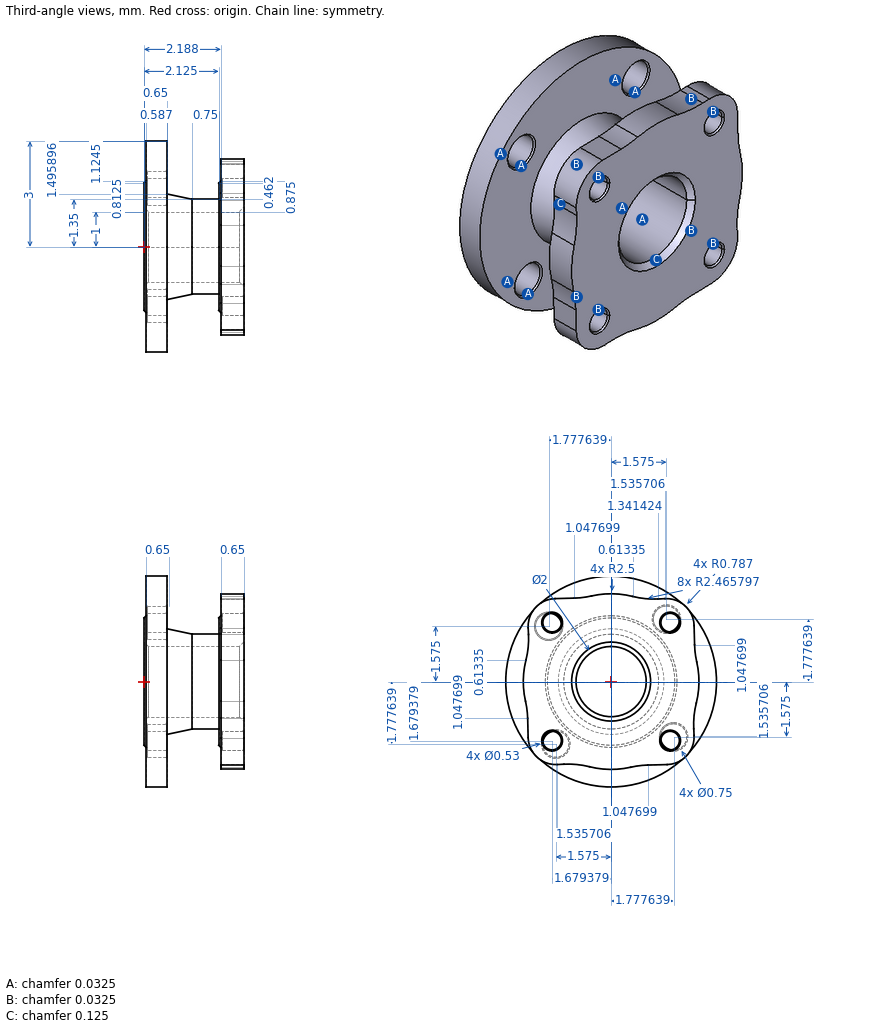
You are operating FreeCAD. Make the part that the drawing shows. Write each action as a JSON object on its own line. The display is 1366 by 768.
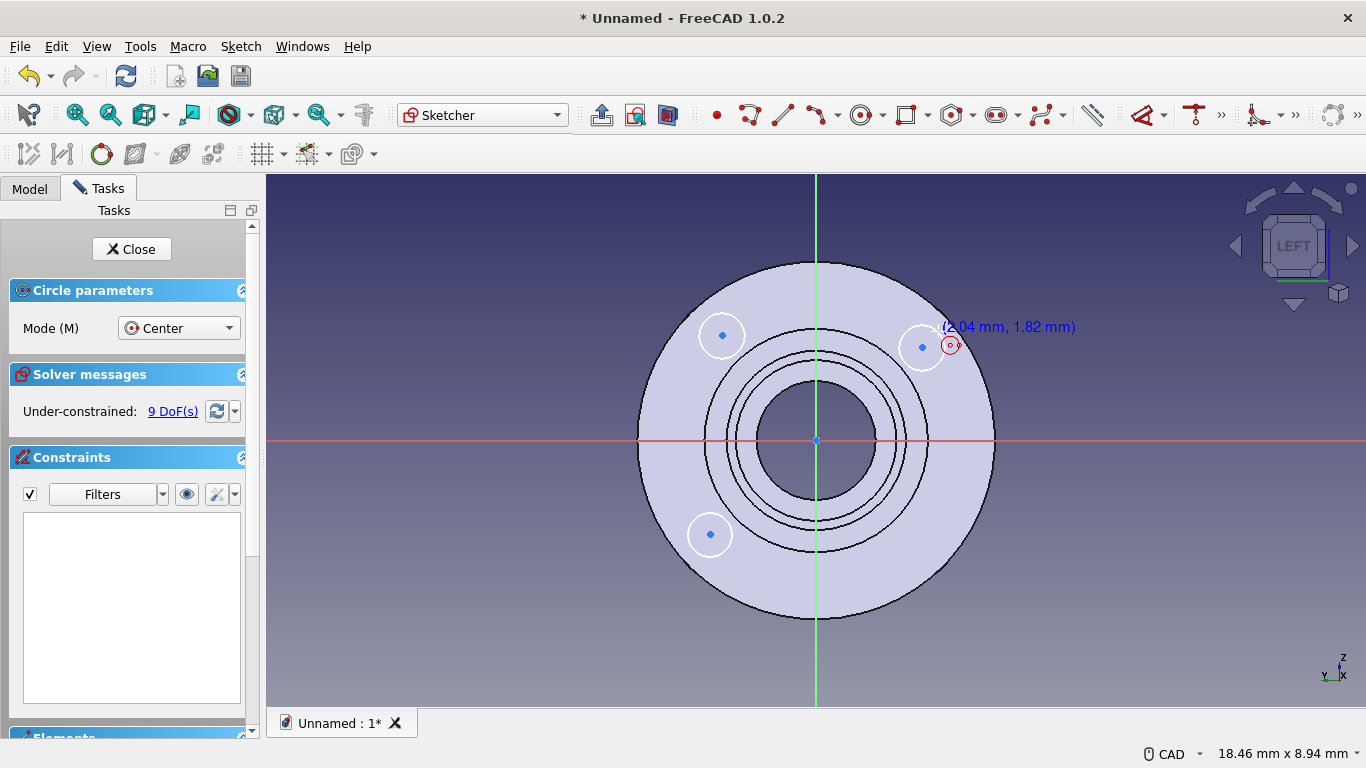
{"action": "left_click", "coordinate": [910, 546]}
{"action": "left_click", "coordinate": [926, 531]}
{"action": "key", "text": "Escape"}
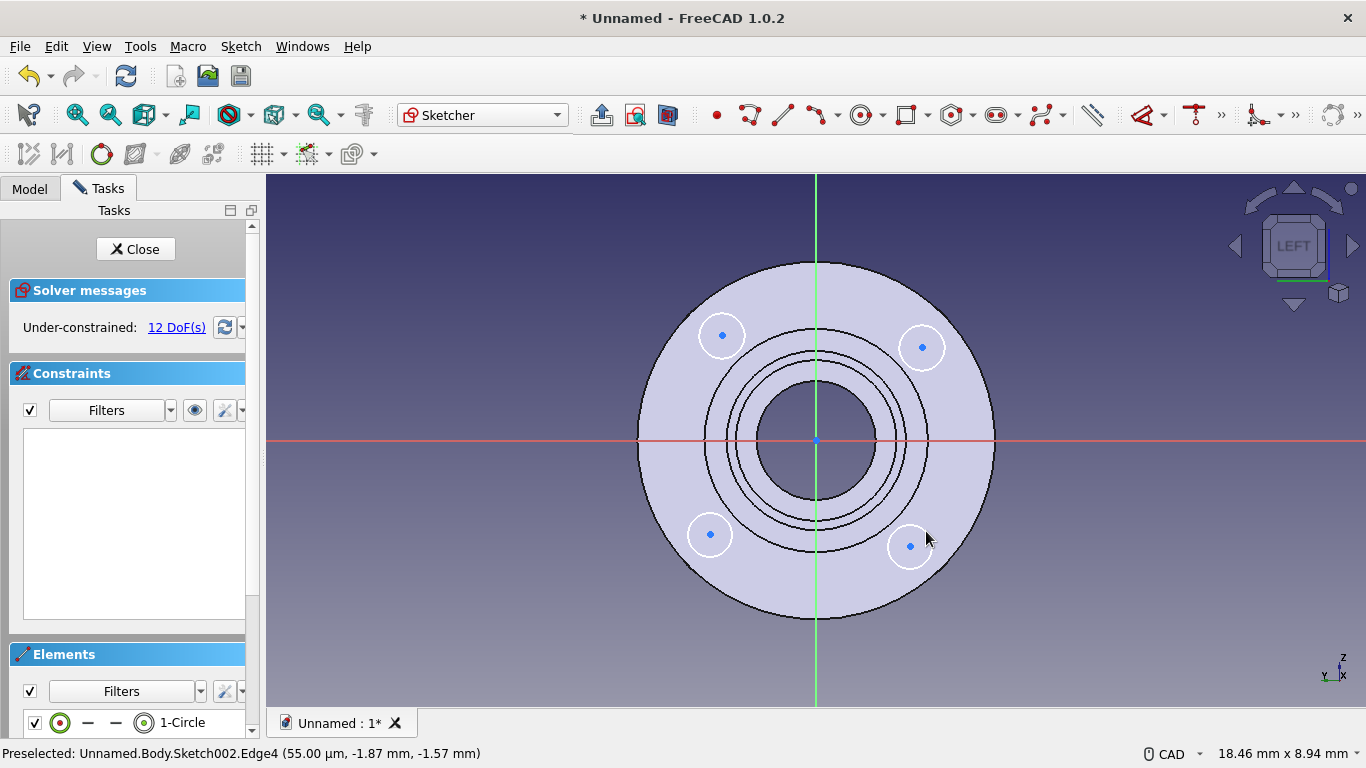
{"action": "left_click", "coordinate": [725, 519]}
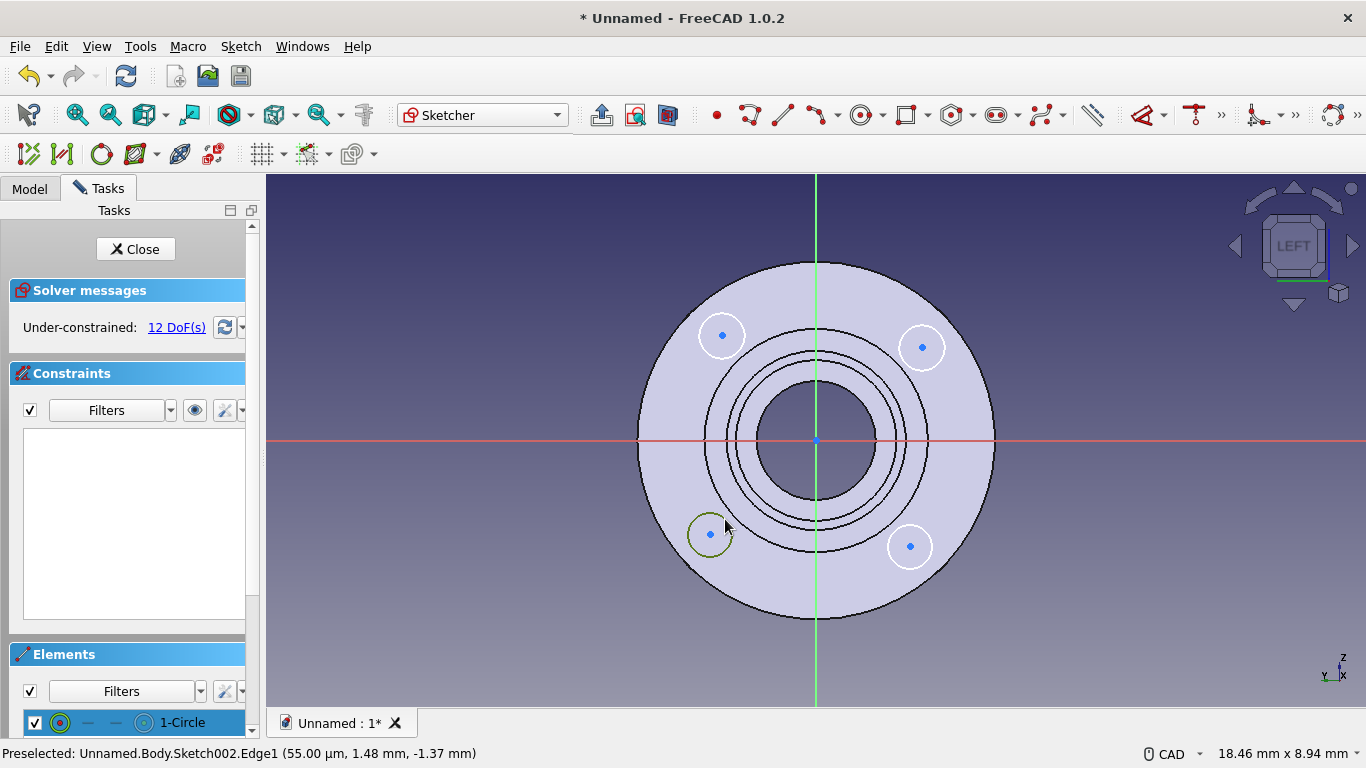
{"action": "left_click", "coordinate": [738, 320]}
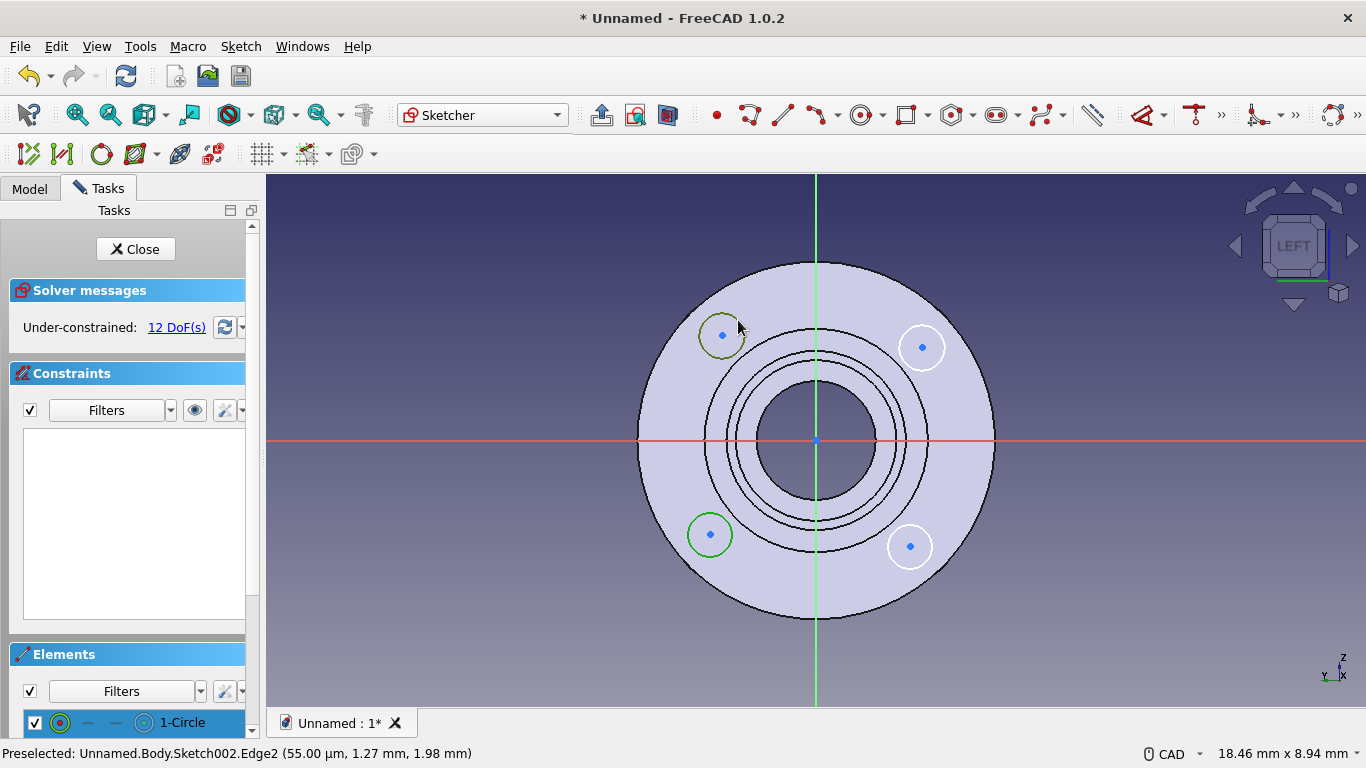
{"action": "left_click", "coordinate": [938, 332]}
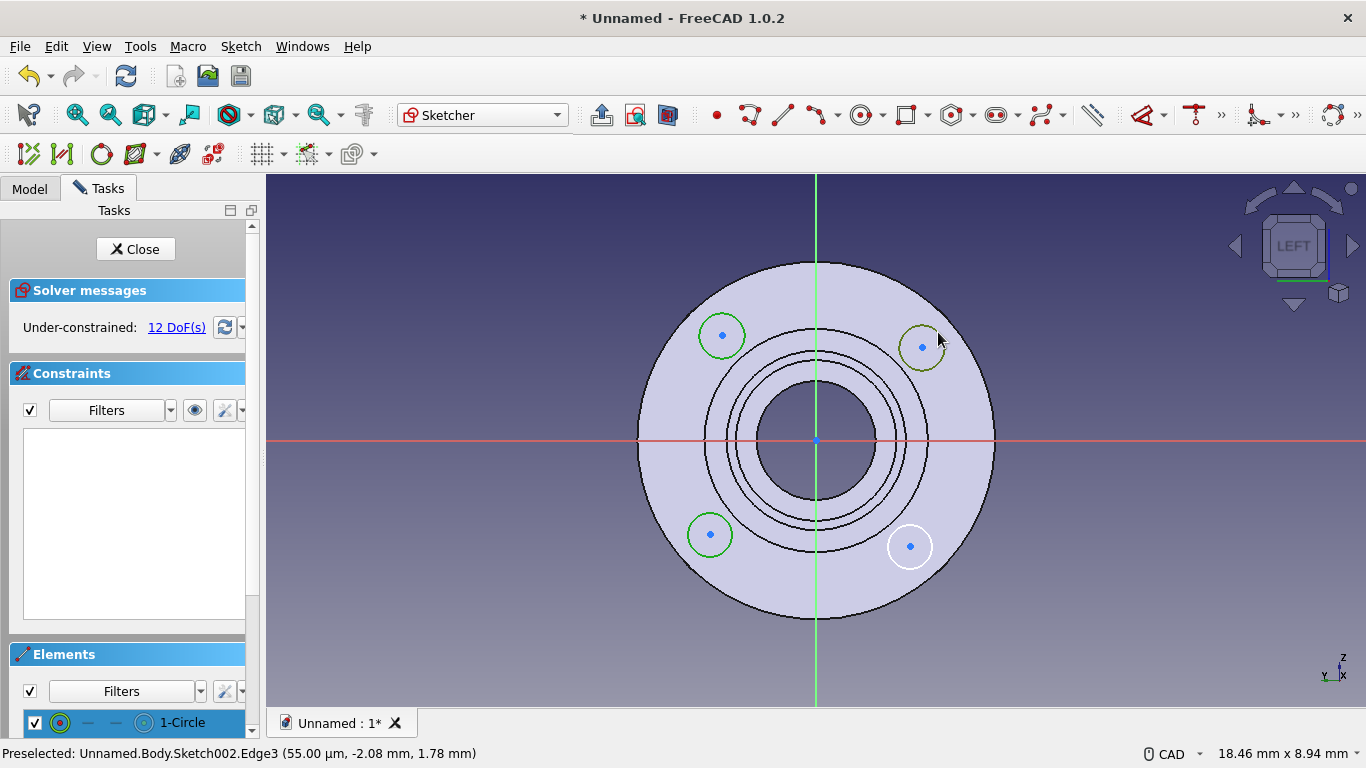
{"action": "left_click", "coordinate": [925, 531]}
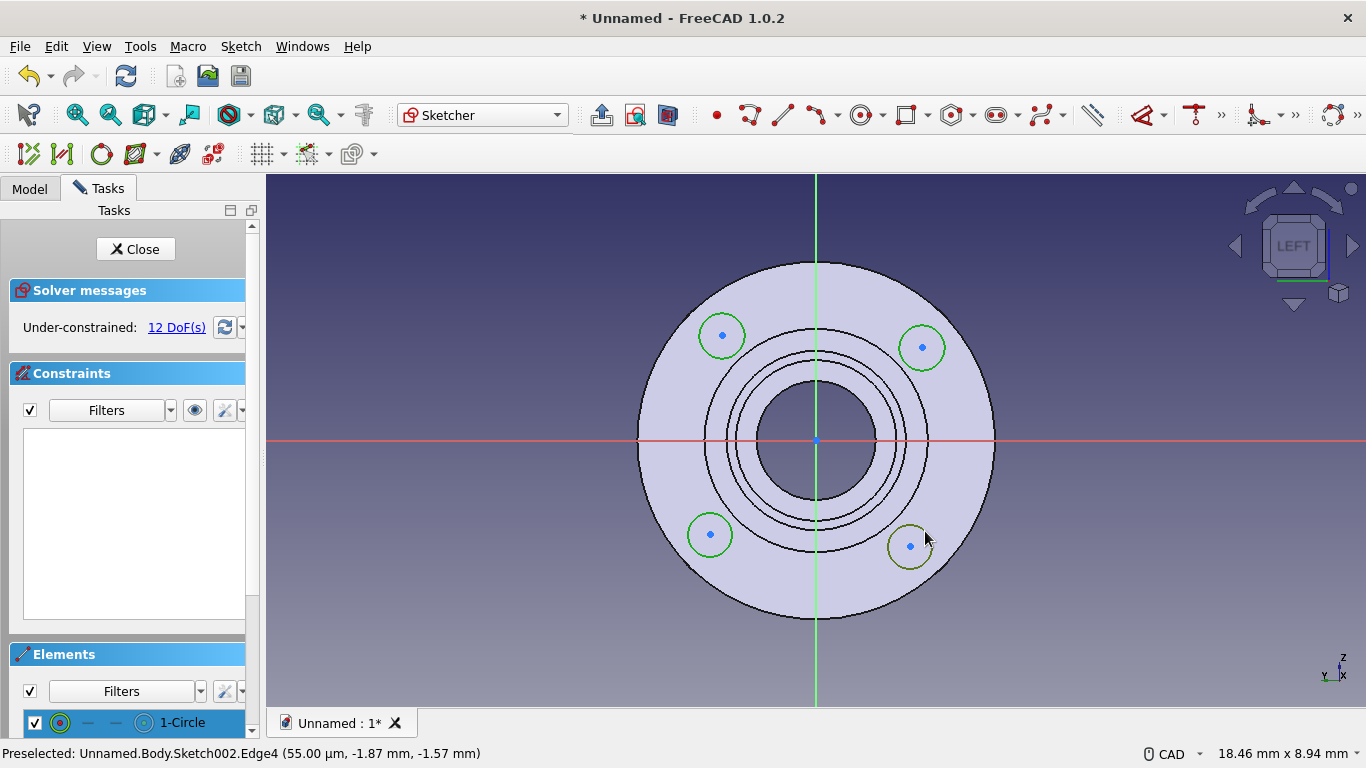
{"action": "key", "text": "e"}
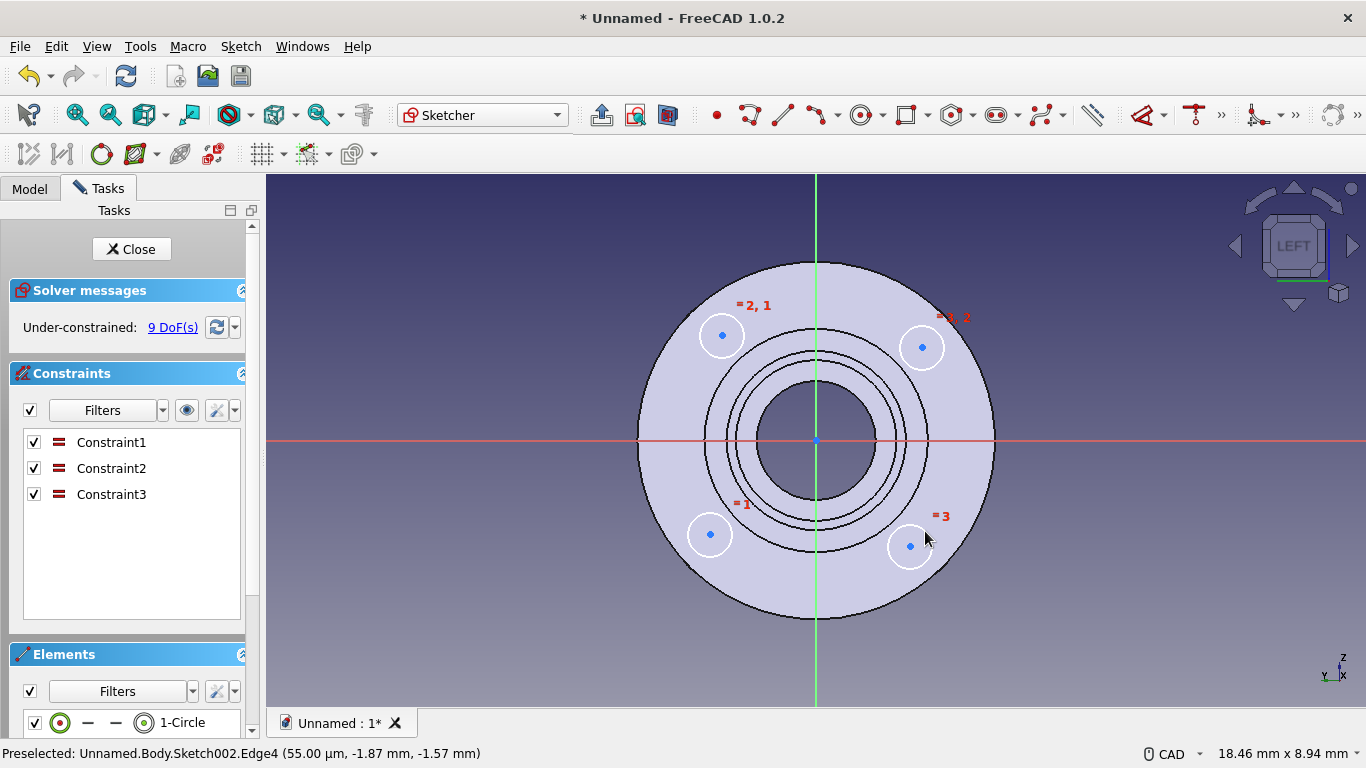
{"action": "key", "text": "d"}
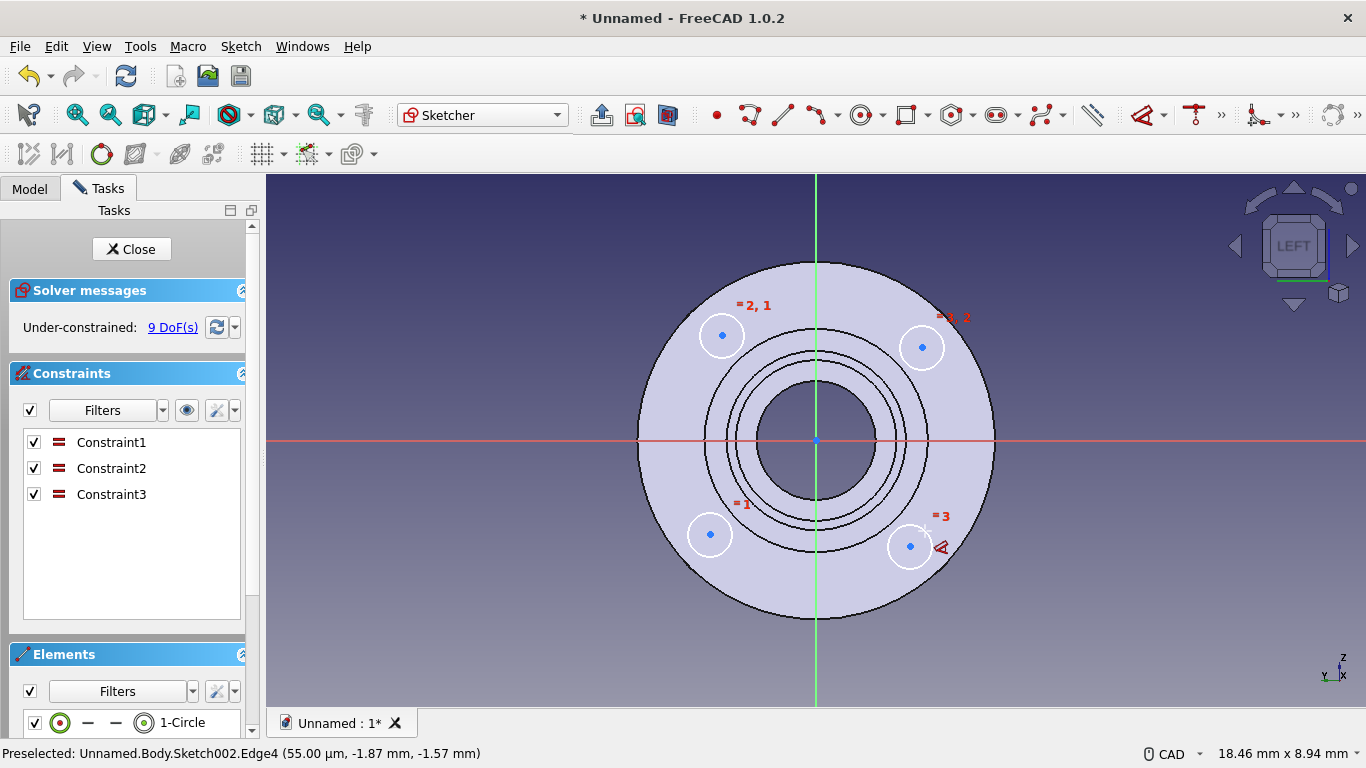
{"action": "left_click", "coordinate": [725, 519]}
{"action": "left_click", "coordinate": [747, 496]}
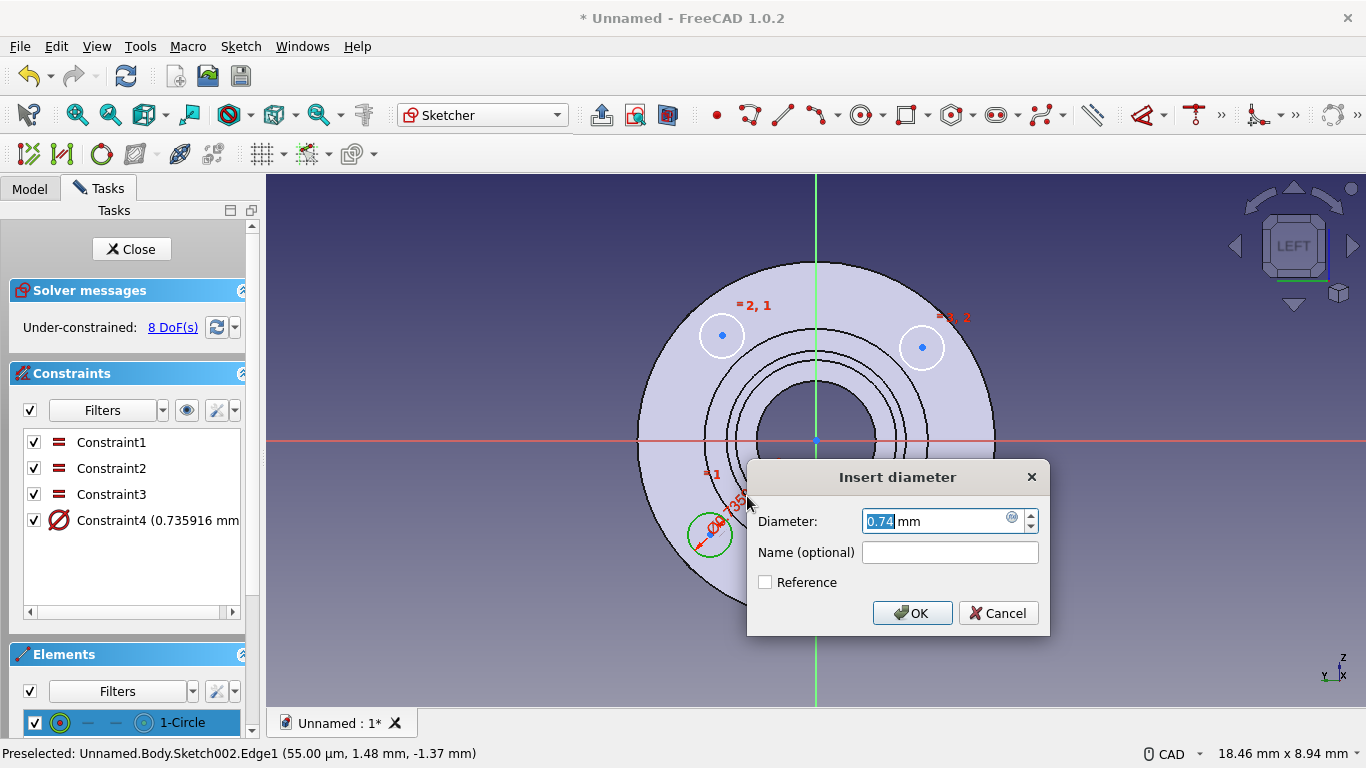
{"action": "type", "text": "0.75"}
{"action": "key", "text": "Return"}